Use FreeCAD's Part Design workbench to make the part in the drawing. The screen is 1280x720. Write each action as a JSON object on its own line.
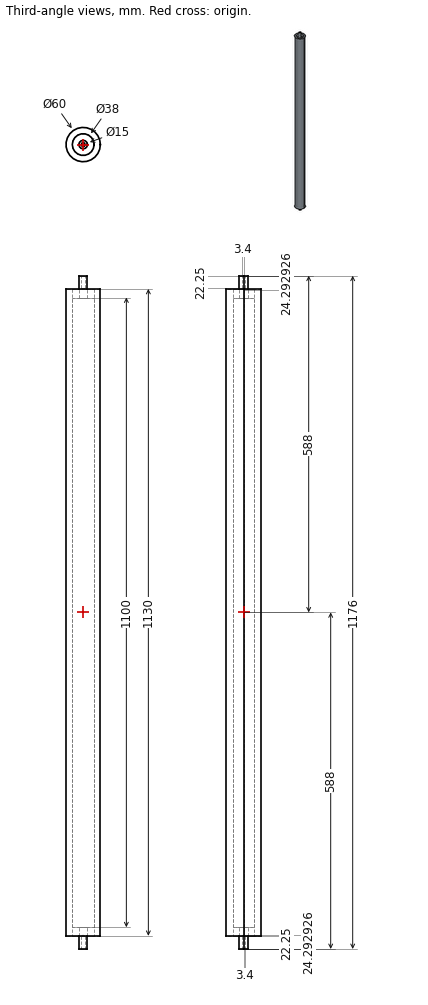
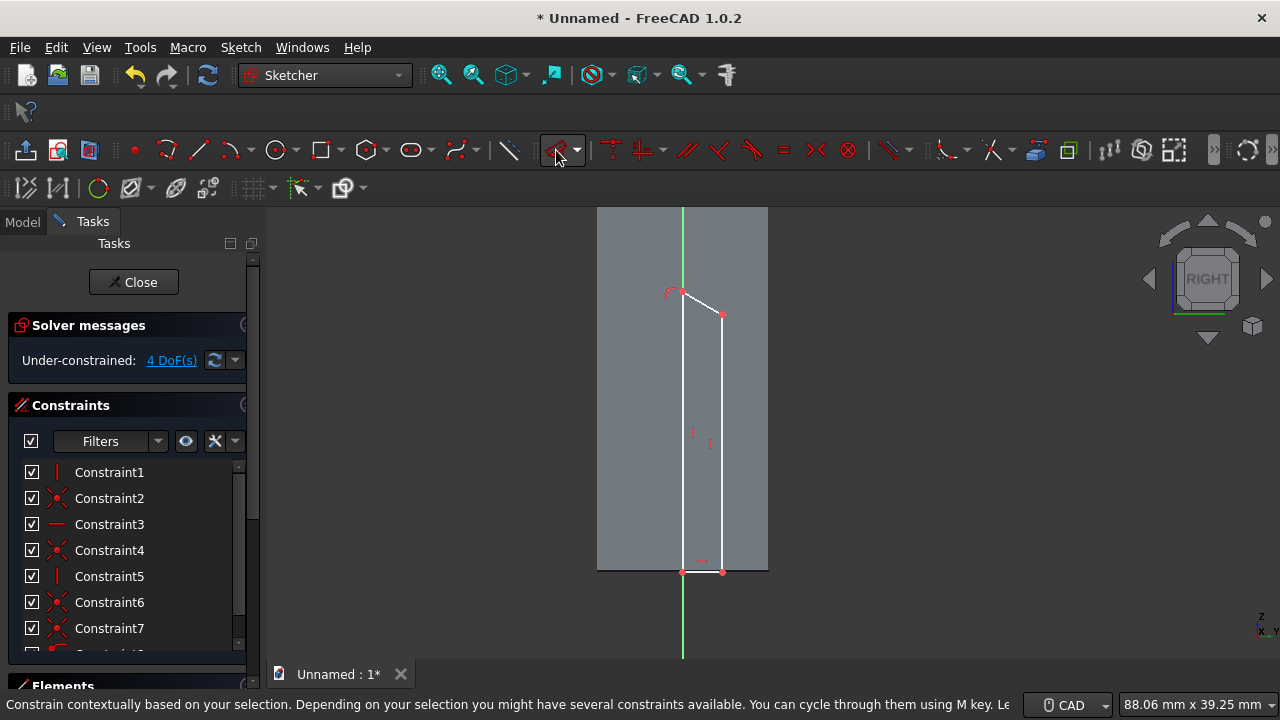
{"action": "left_click", "coordinate": [694, 572]}
{"action": "left_click", "coordinate": [702, 606]}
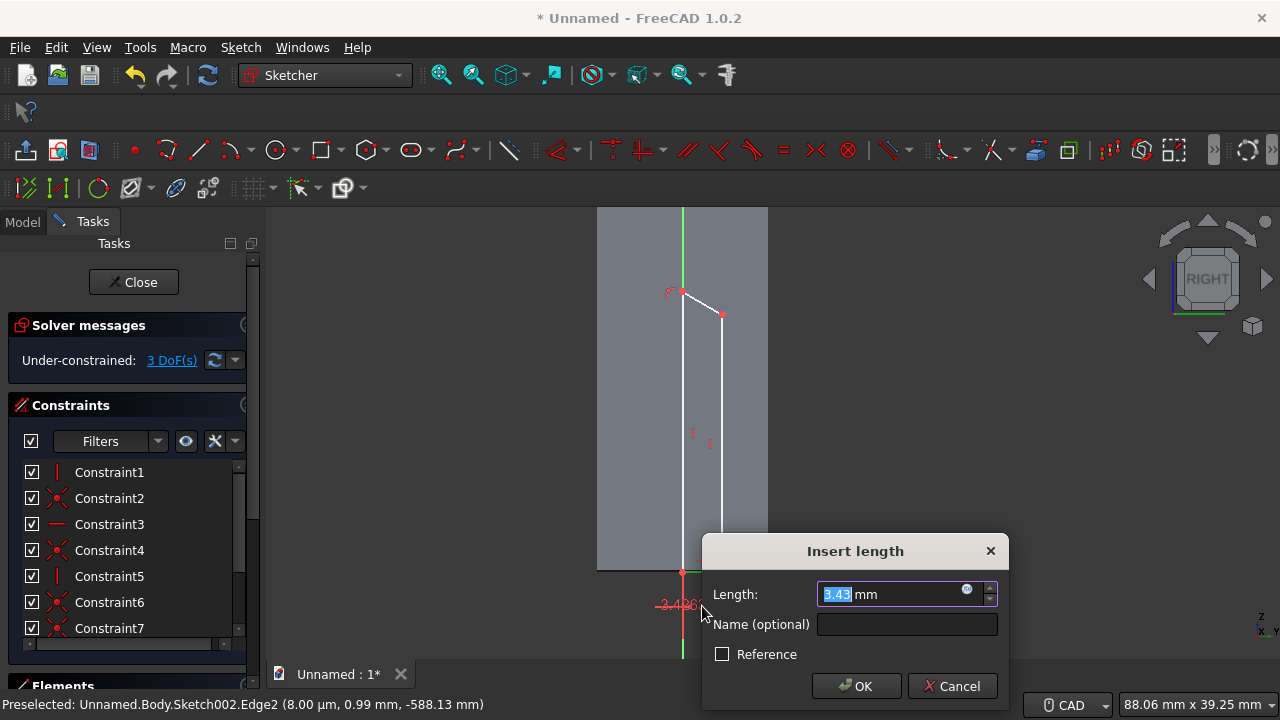
{"action": "type", "text": "3.4"}
{"action": "key", "text": "Return"}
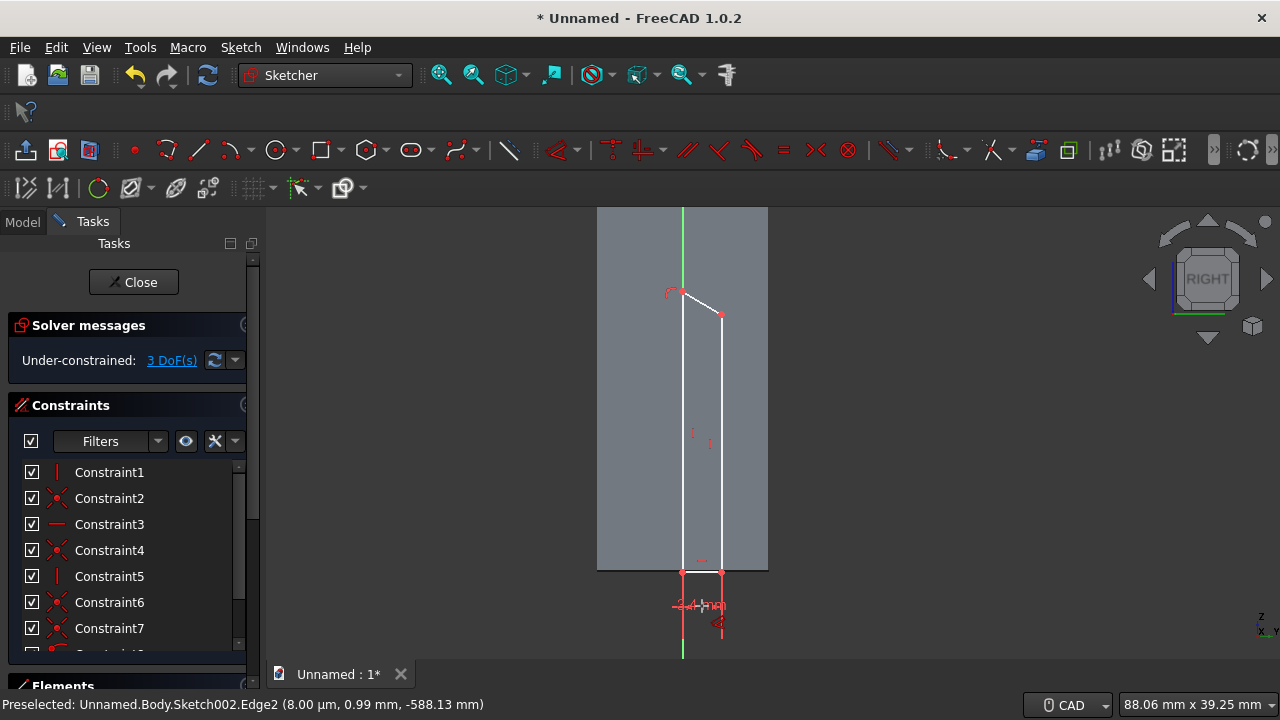
{"action": "left_click", "coordinate": [683, 572]}
{"action": "left_click", "coordinate": [649, 404]}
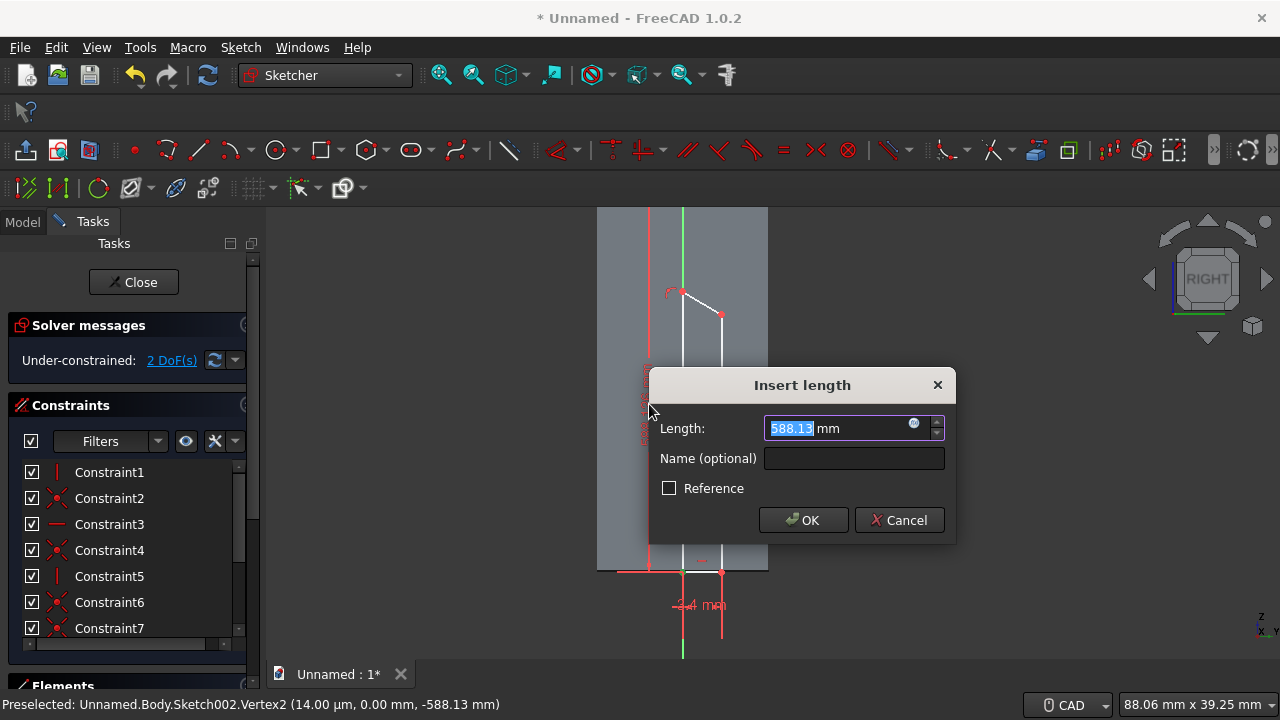
{"action": "type", "text": "588"}
{"action": "key", "text": "Return"}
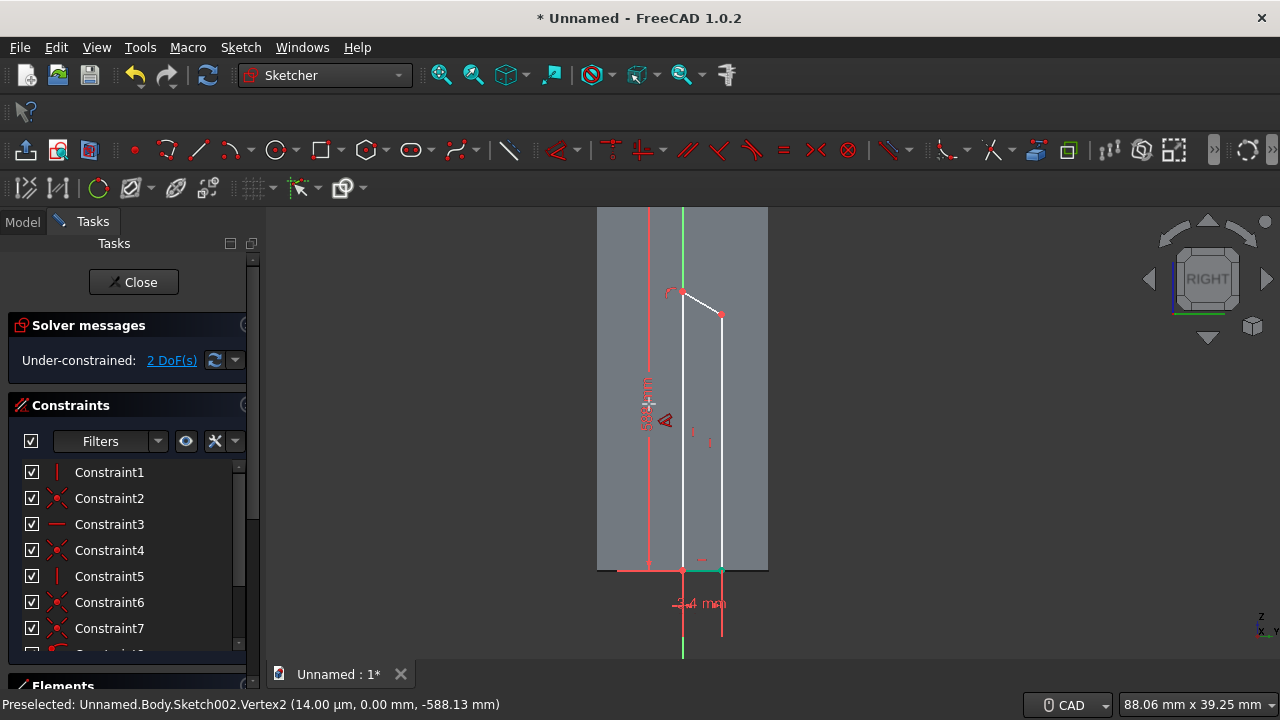
{"action": "left_click", "coordinate": [722, 494]}
{"action": "left_click", "coordinate": [756, 443]}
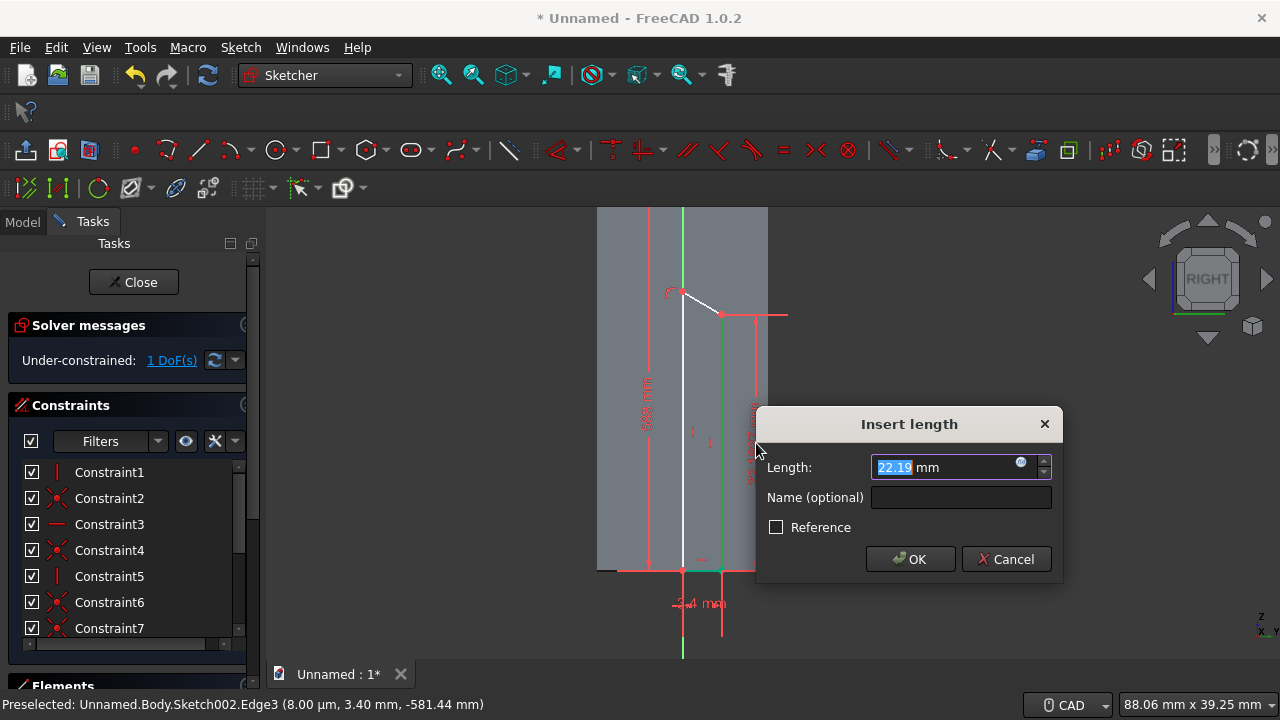
{"action": "type", "text": "22.25"}
{"action": "key", "text": "Return"}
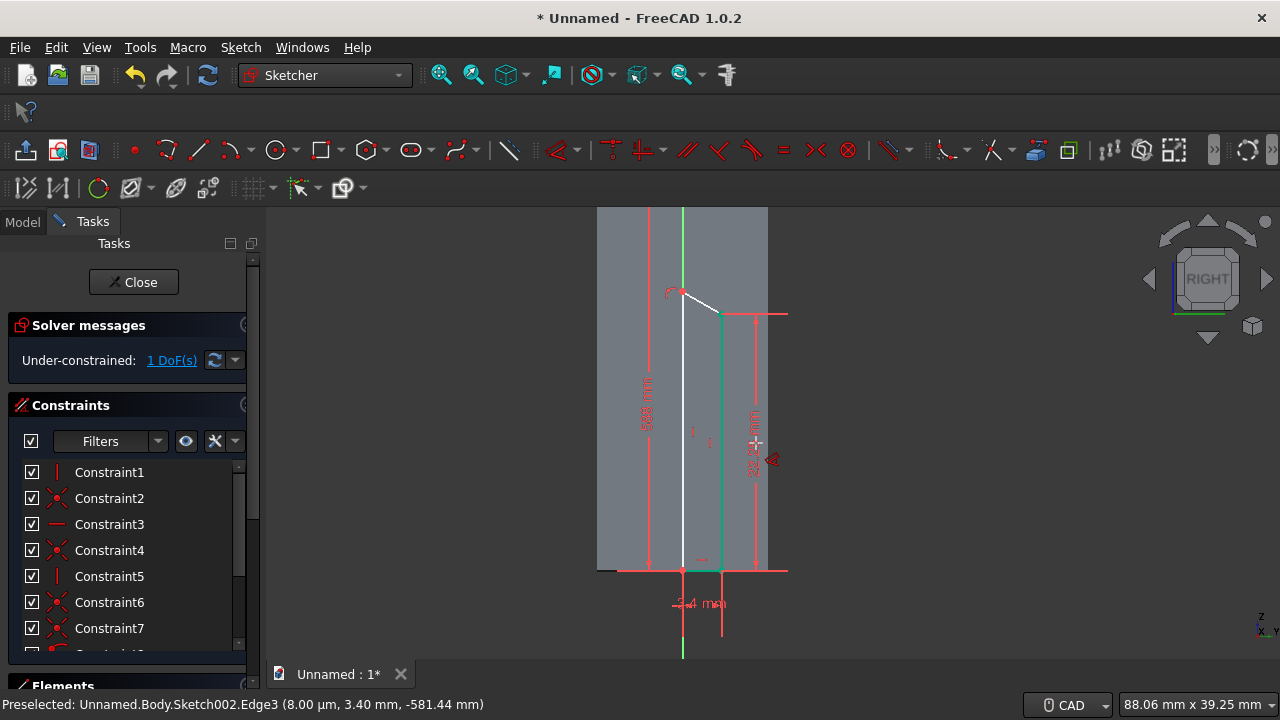
{"action": "left_click", "coordinate": [683, 376]}
{"action": "left_click", "coordinate": [649, 431]}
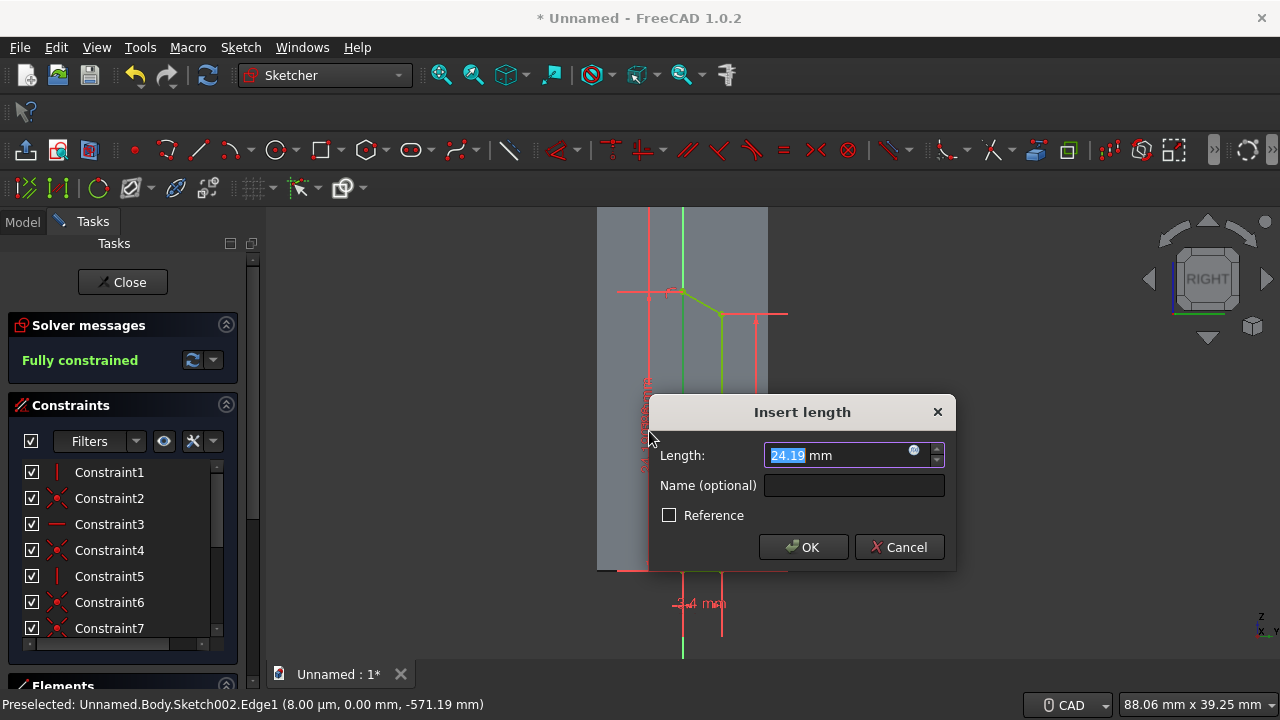
{"action": "type", "text": "24.292926"}
{"action": "key", "text": "Return"}
{"action": "key", "text": "Escape"}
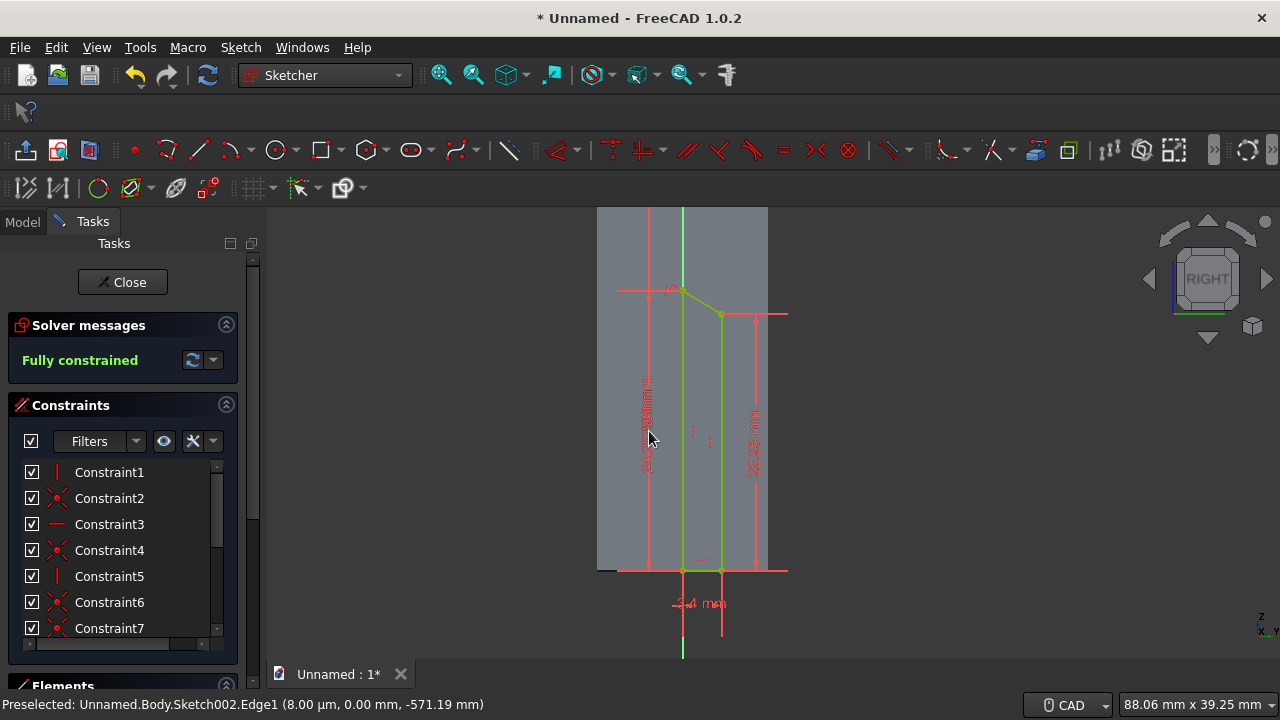
{"action": "left_click", "coordinate": [123, 282]}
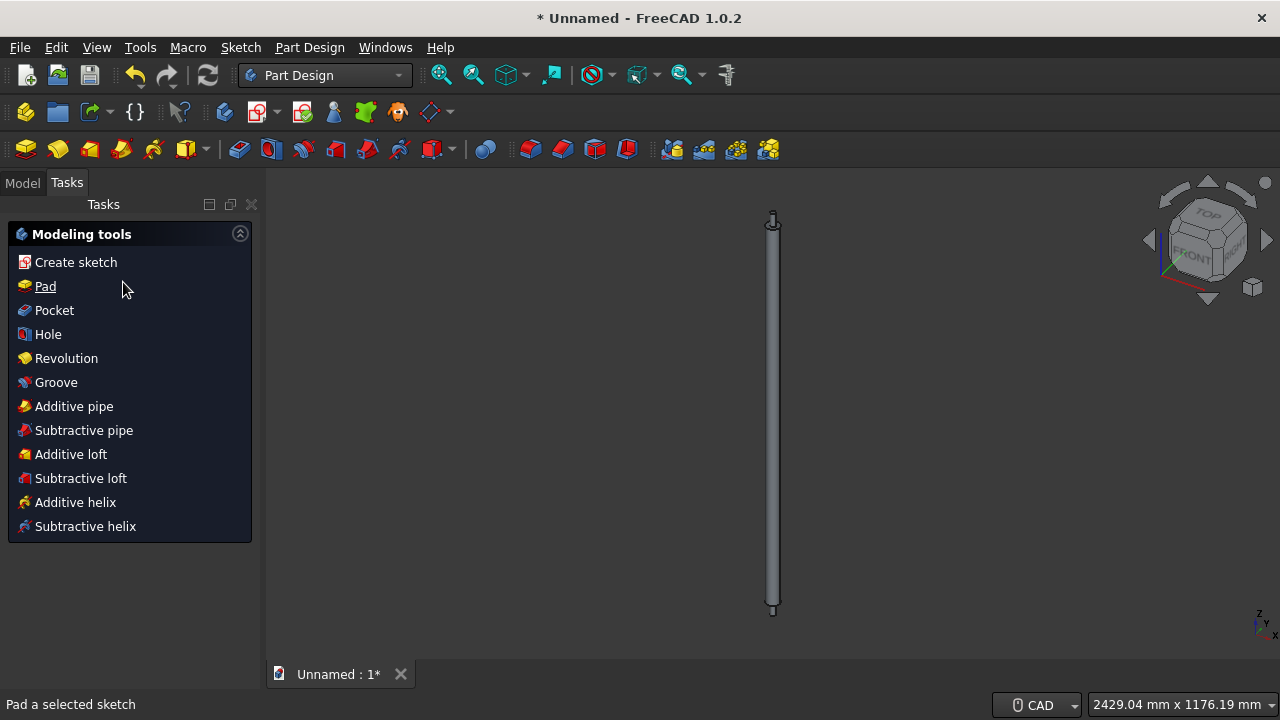
{"action": "left_click", "coordinate": [304, 150]}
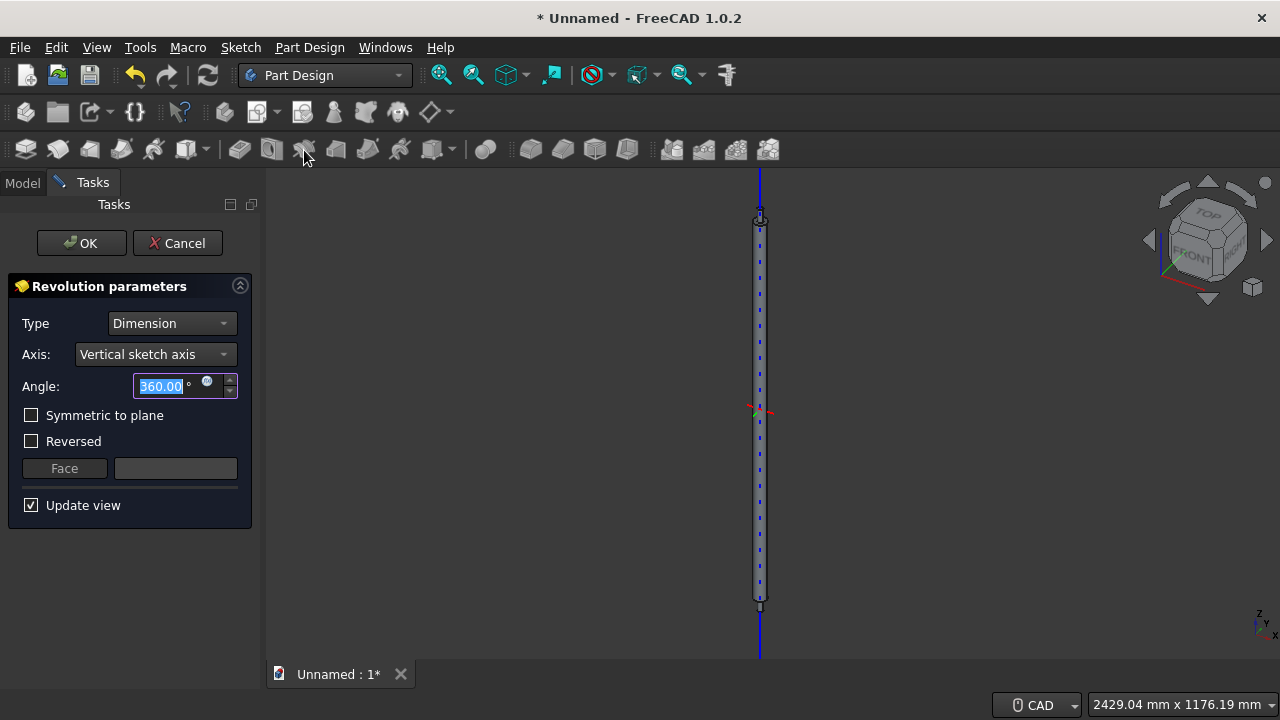
{"action": "left_click", "coordinate": [82, 243]}